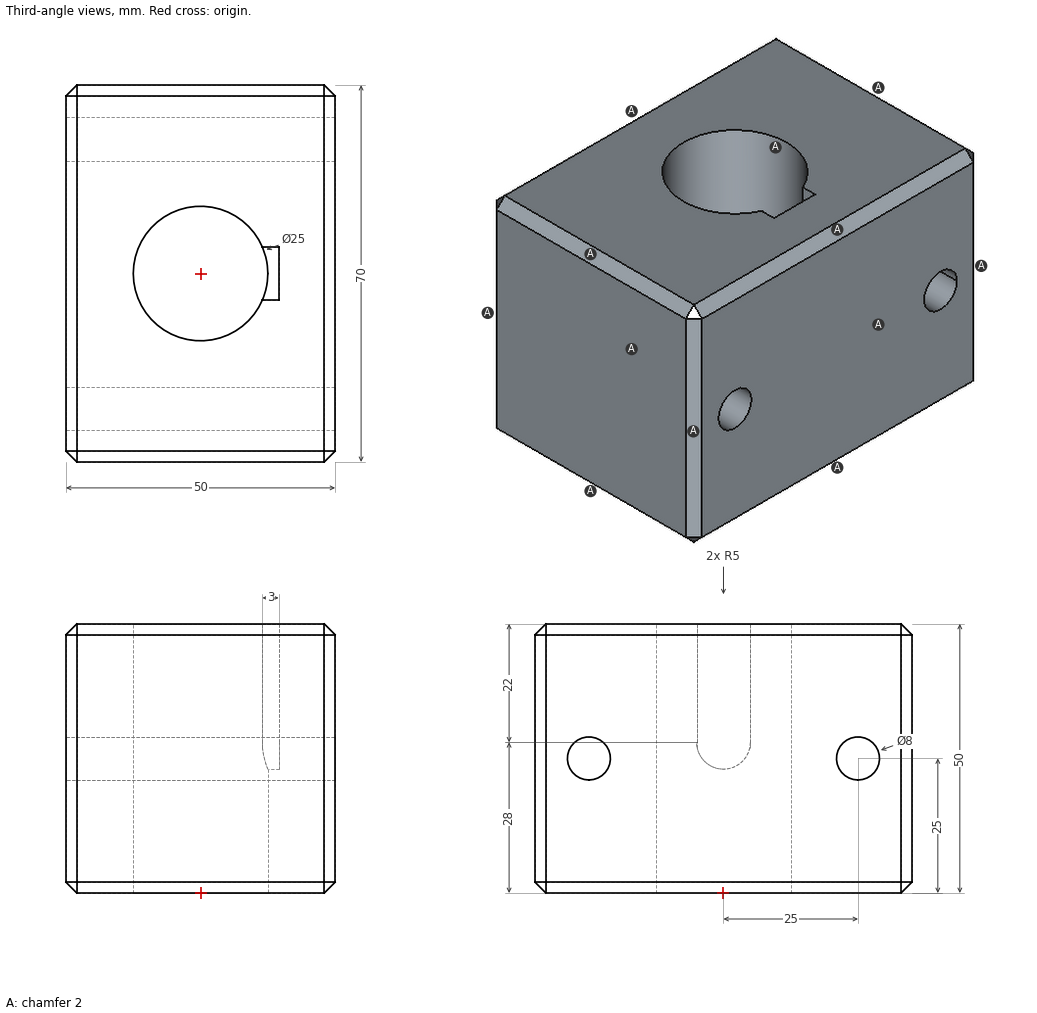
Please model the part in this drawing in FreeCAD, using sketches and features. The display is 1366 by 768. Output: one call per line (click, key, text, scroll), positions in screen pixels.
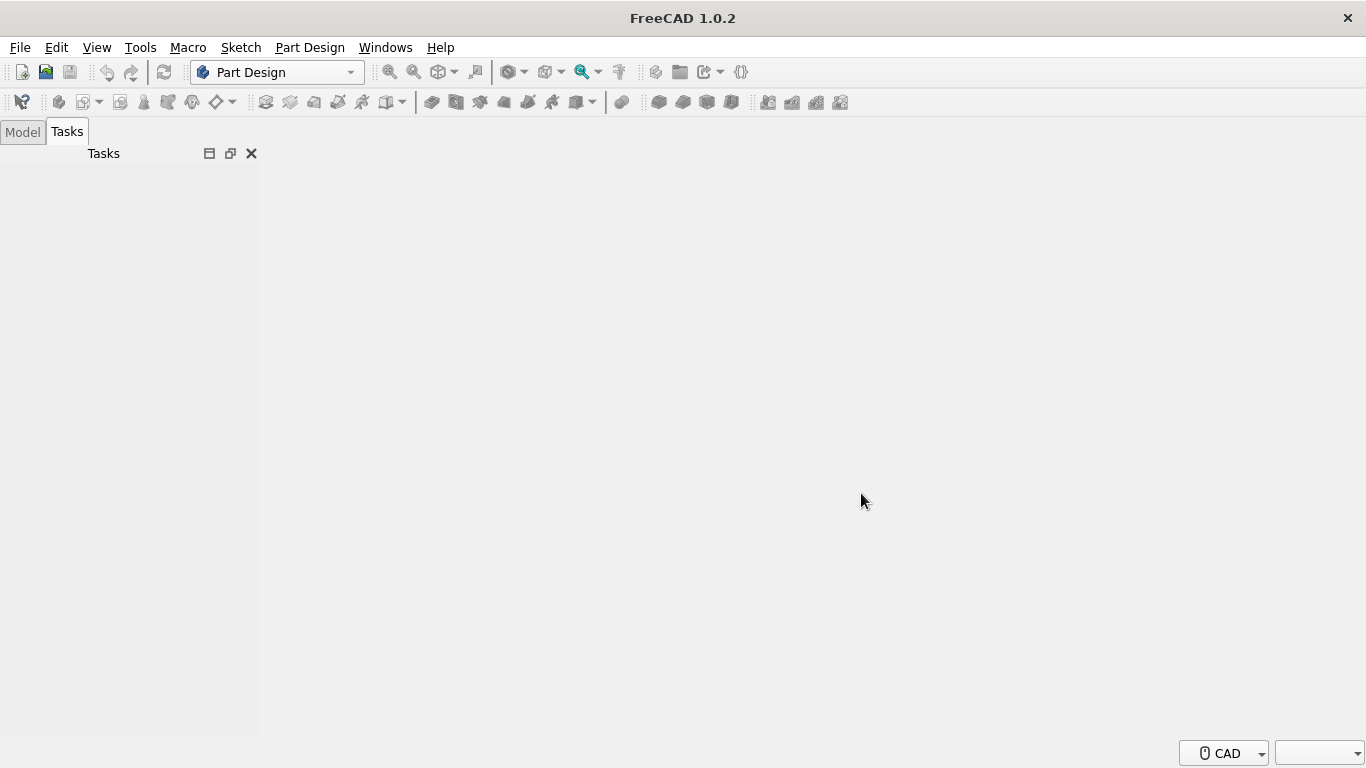
click(22, 72)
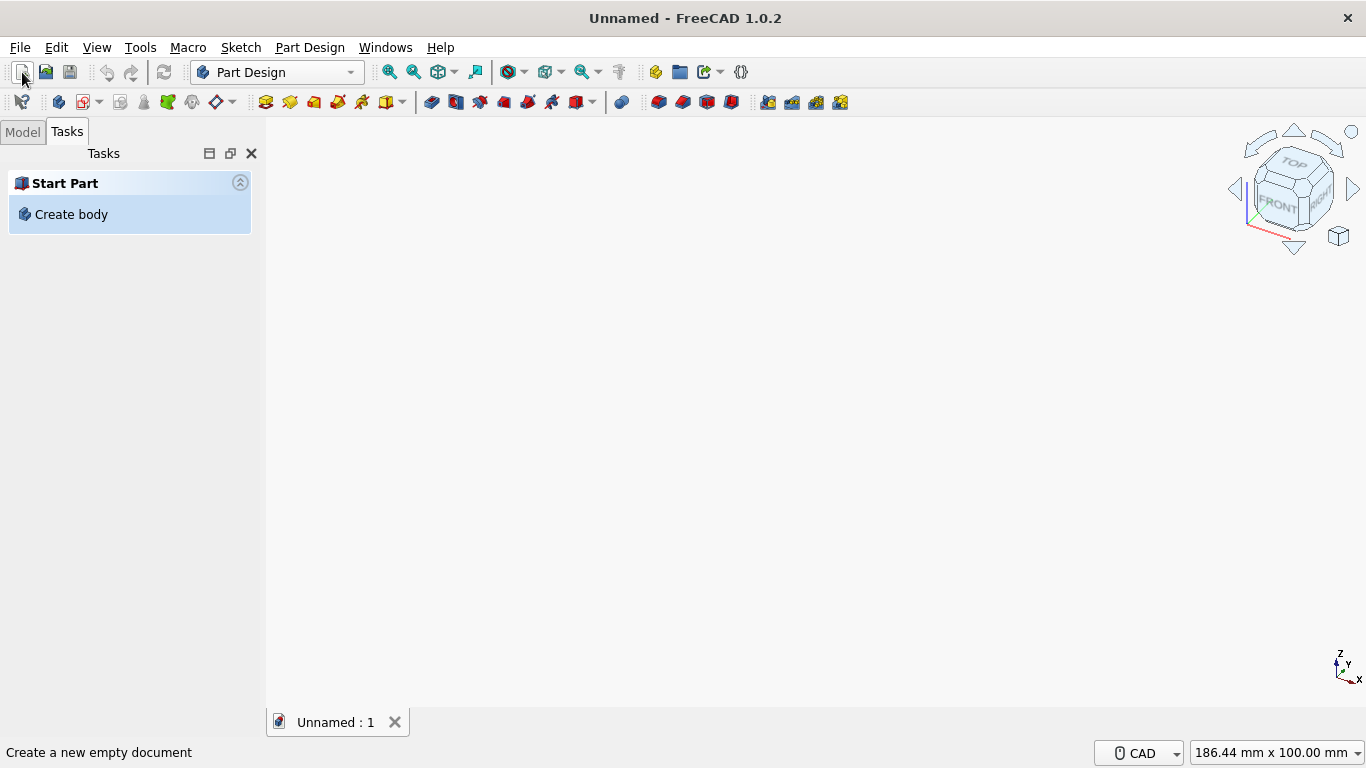
click(84, 102)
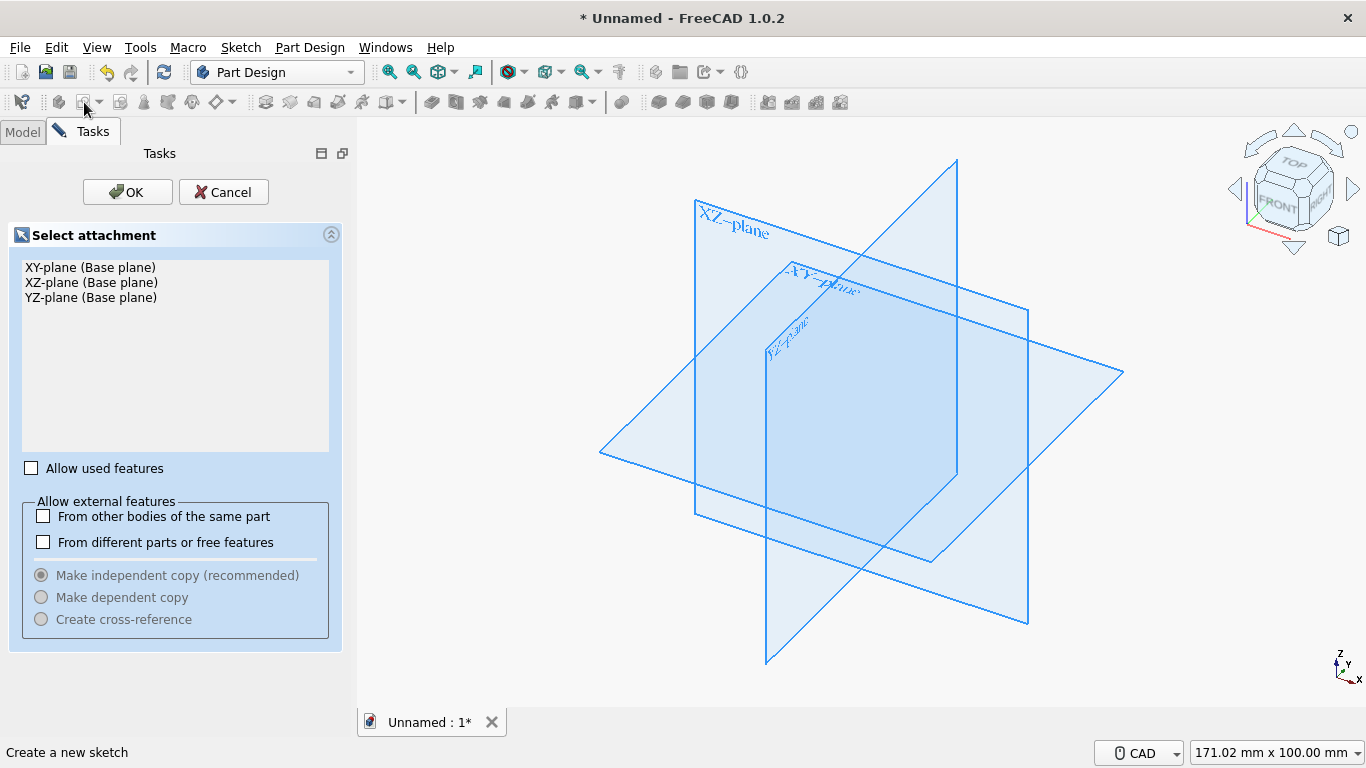
click(82, 268)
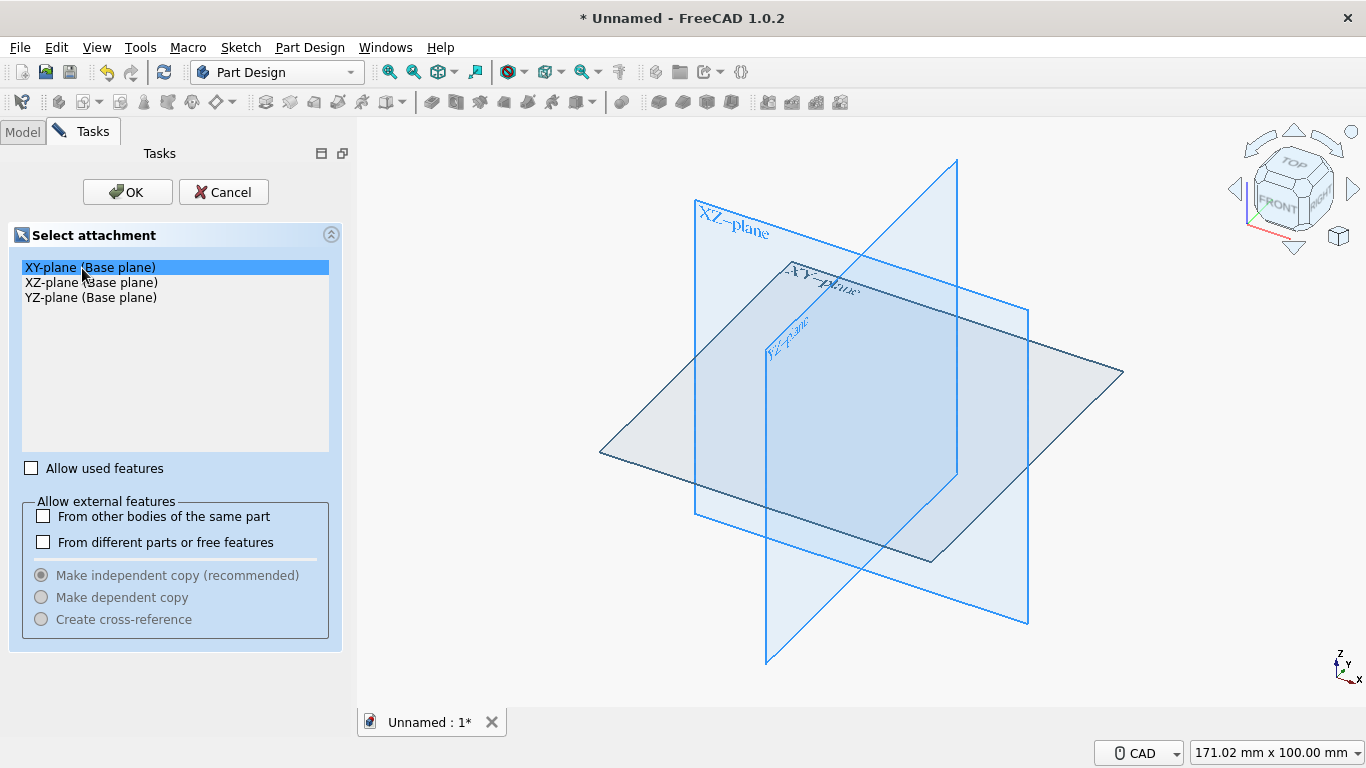
click(128, 192)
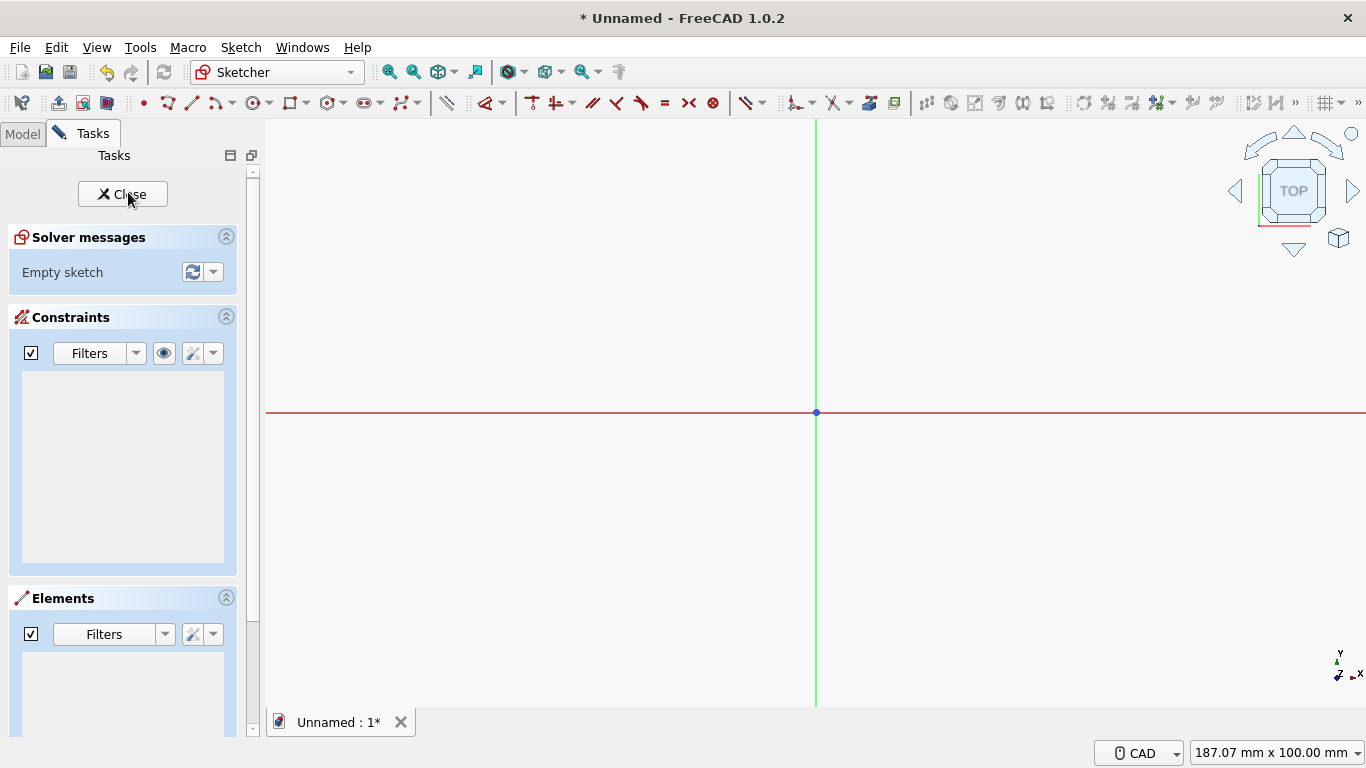
click(308, 104)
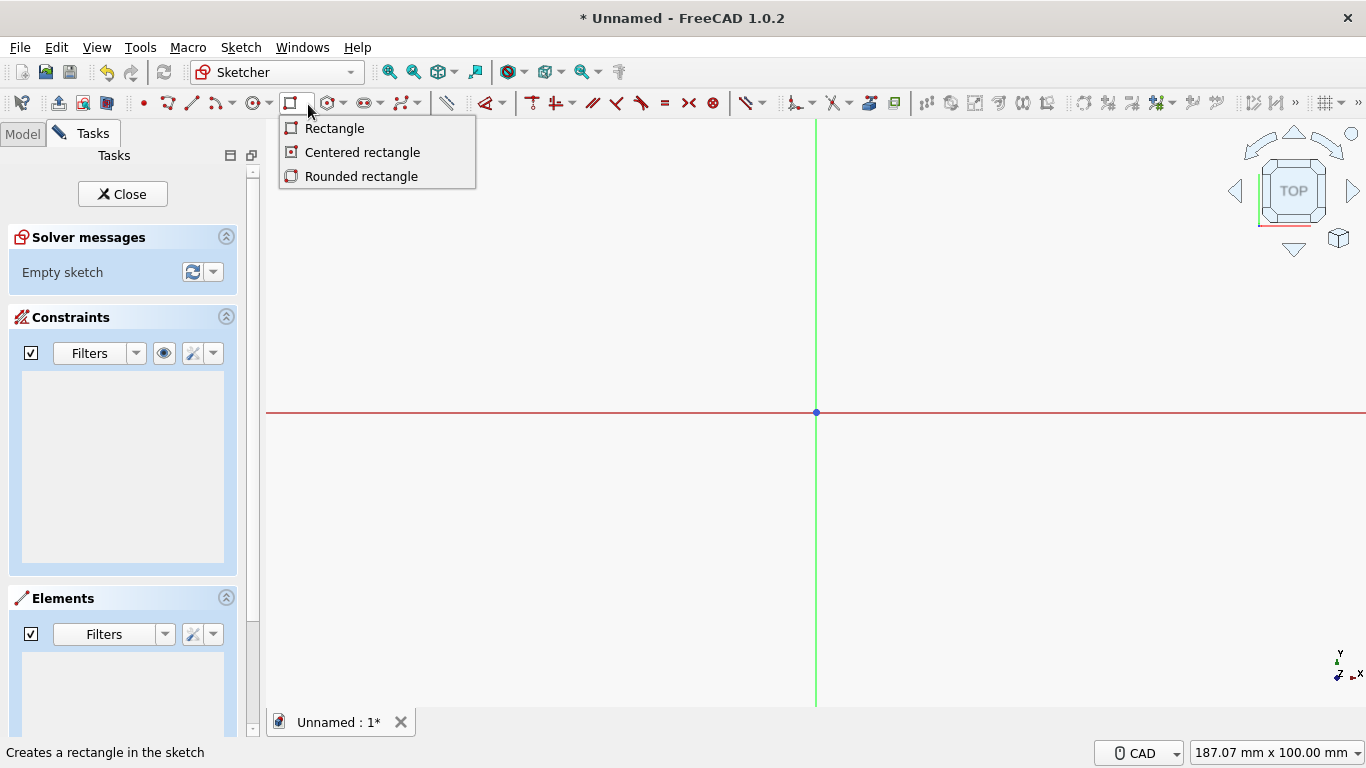
click(378, 152)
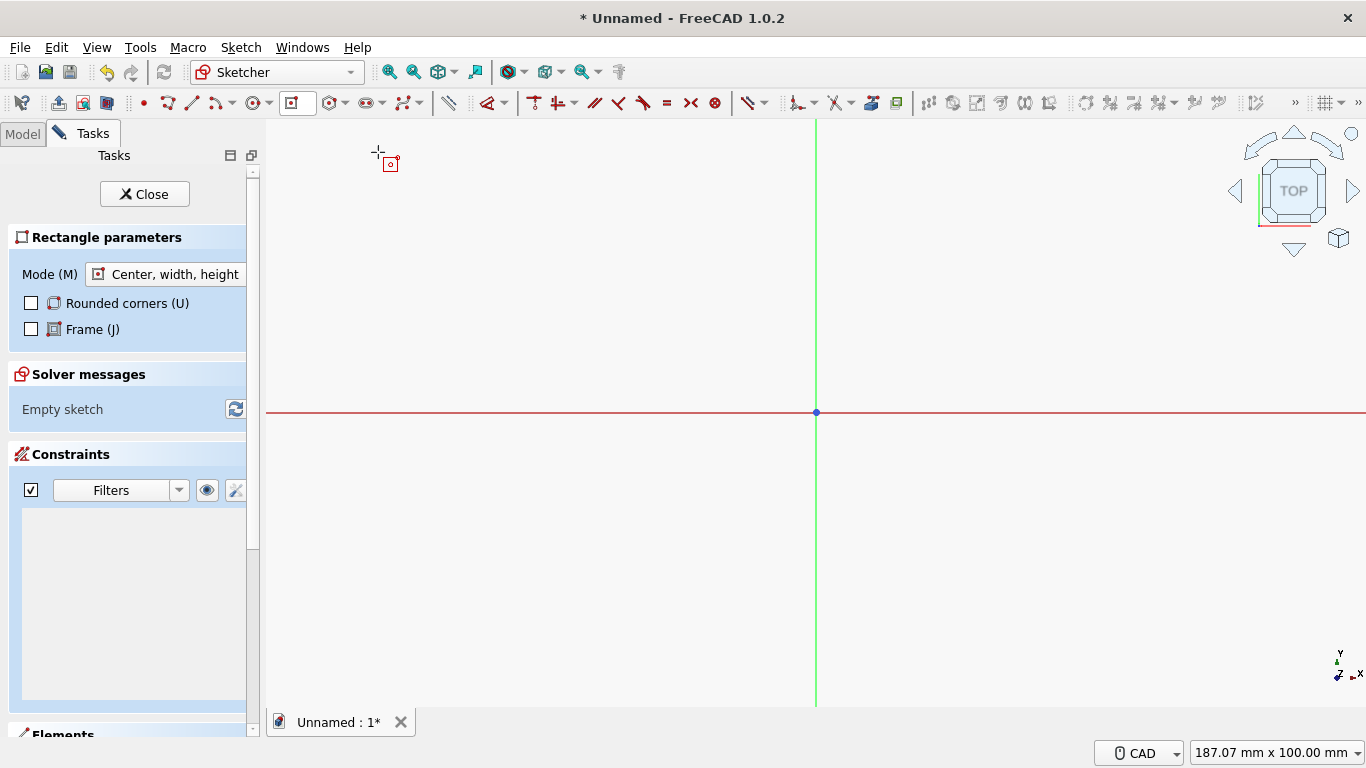
click(816, 413)
move(963, 207)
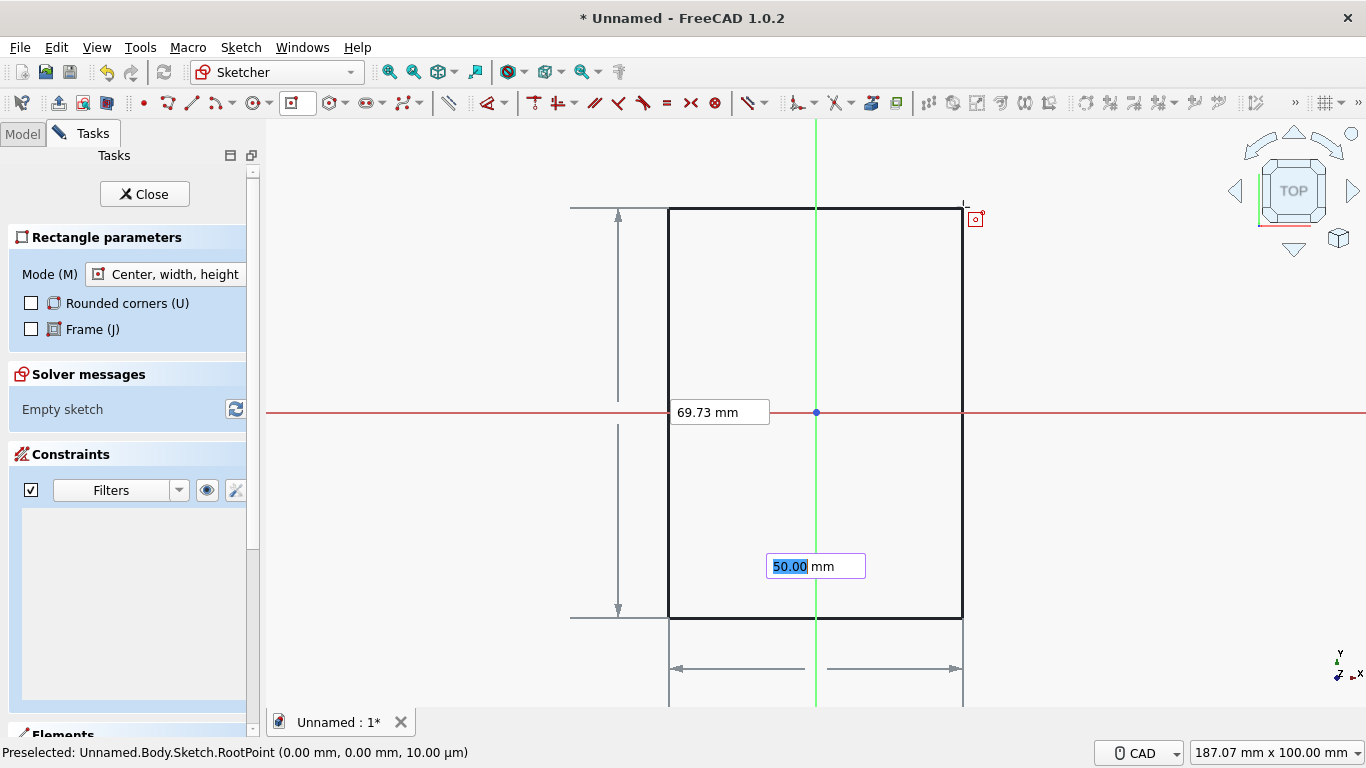
text(50)
key(Tab)
text(70)
key(Return)
key(Escape)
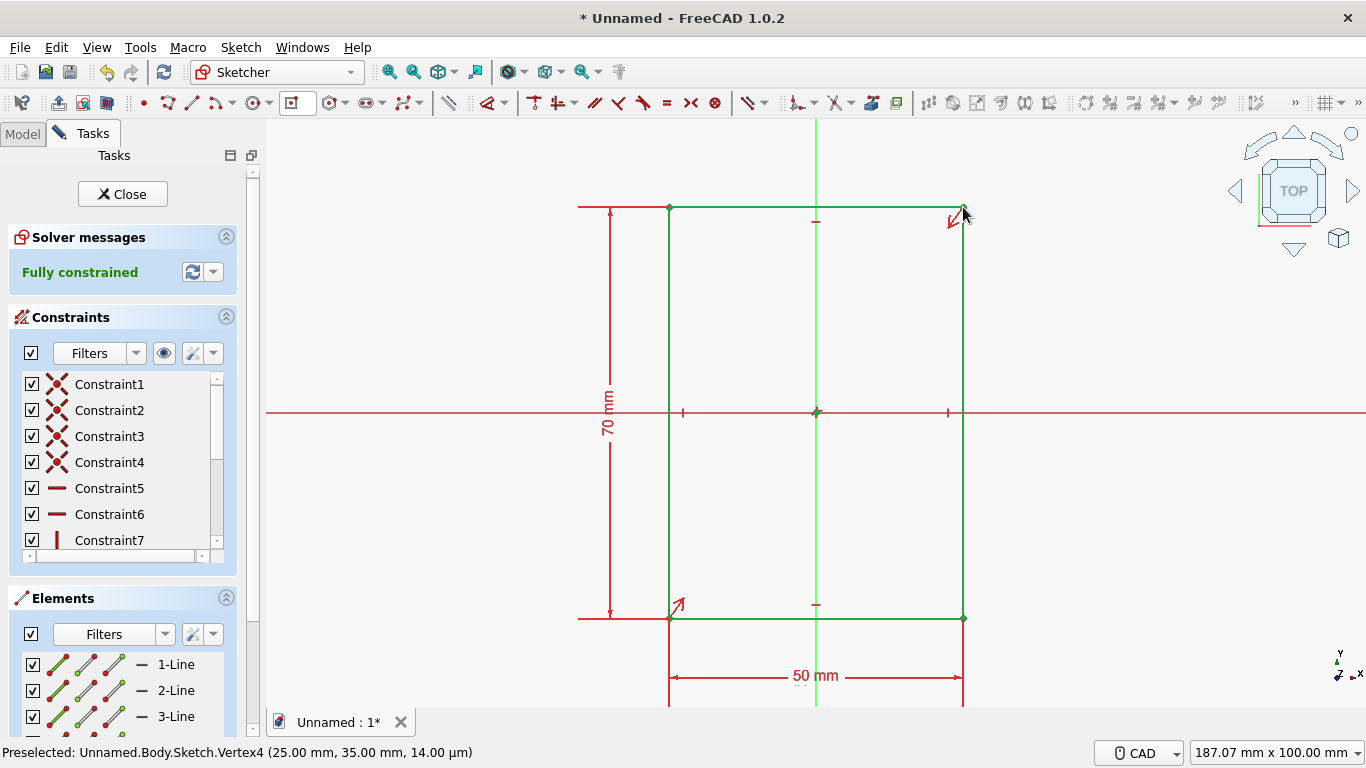
click(123, 194)